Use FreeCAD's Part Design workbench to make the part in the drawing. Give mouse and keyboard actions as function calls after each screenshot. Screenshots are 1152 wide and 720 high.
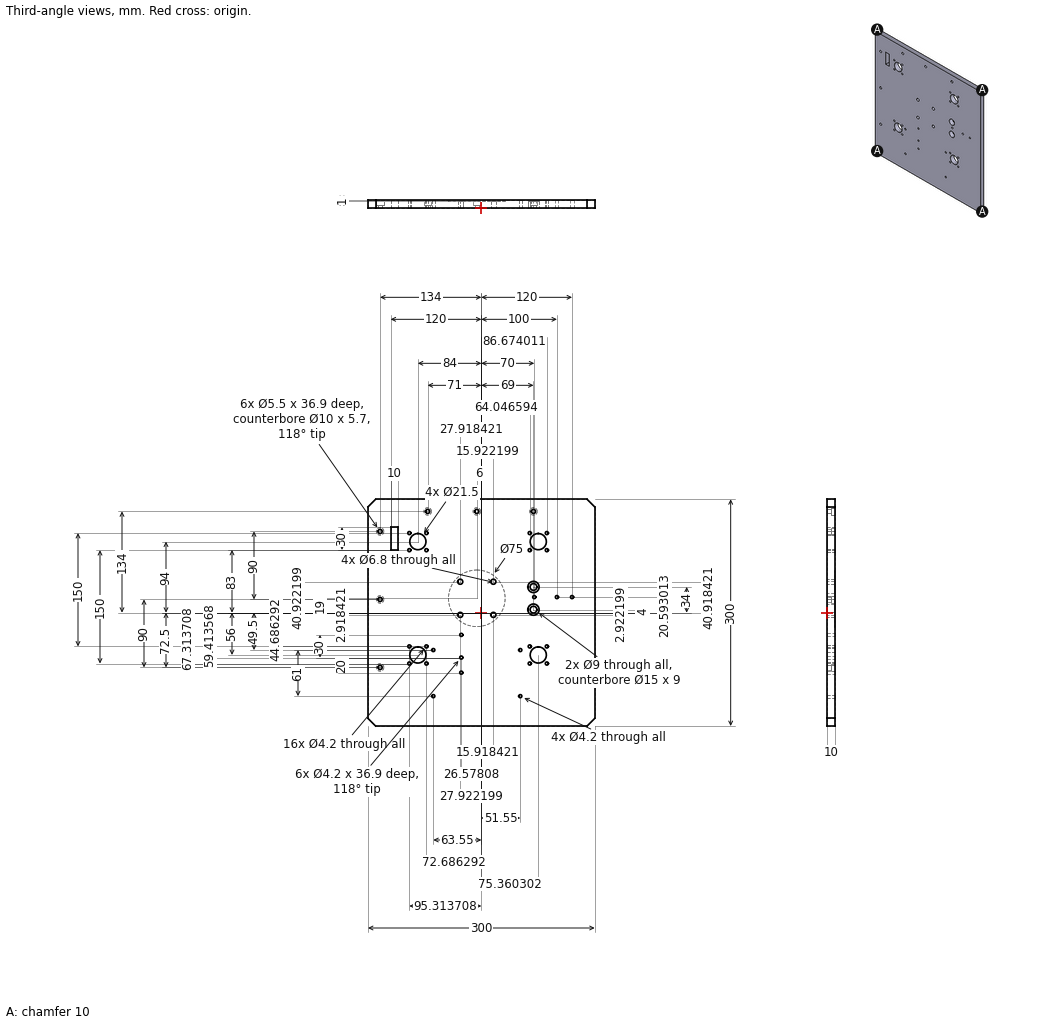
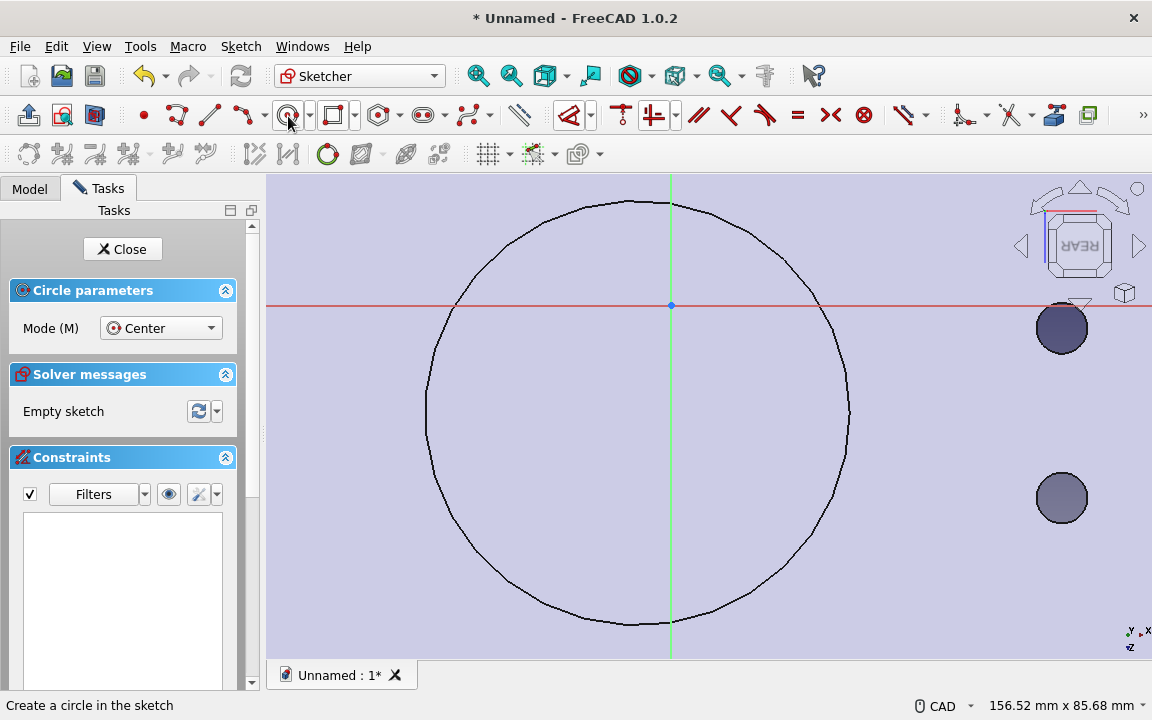
click(762, 537)
move(775, 524)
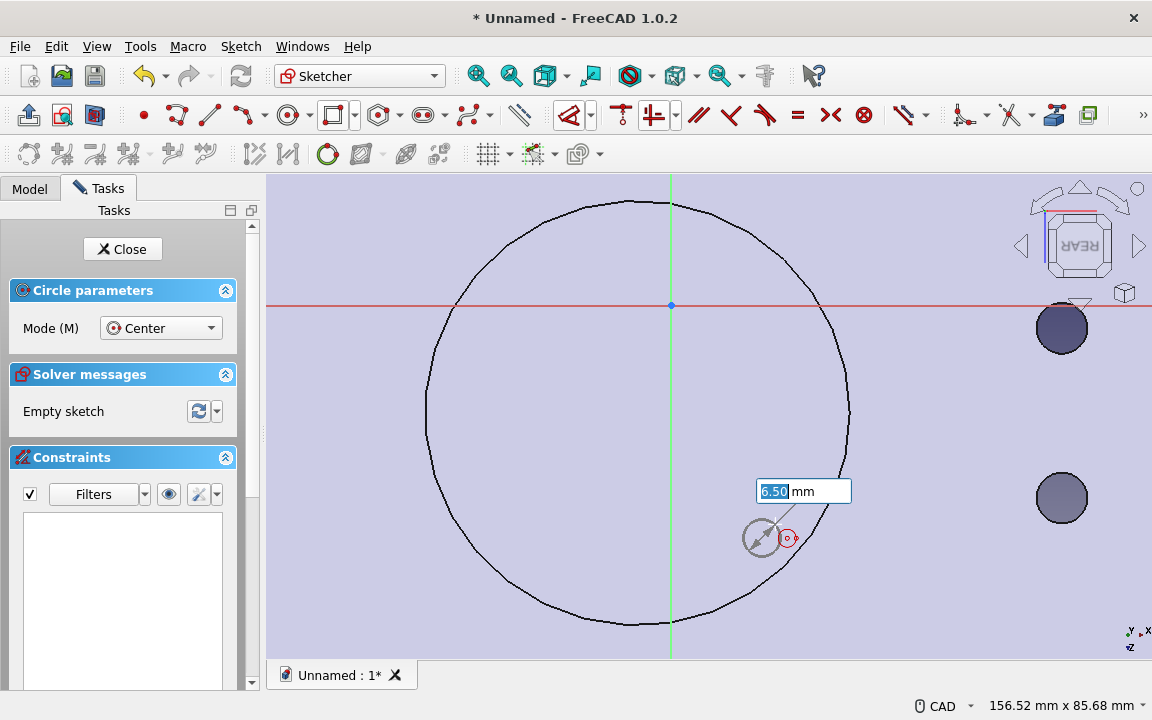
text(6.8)
key(Return)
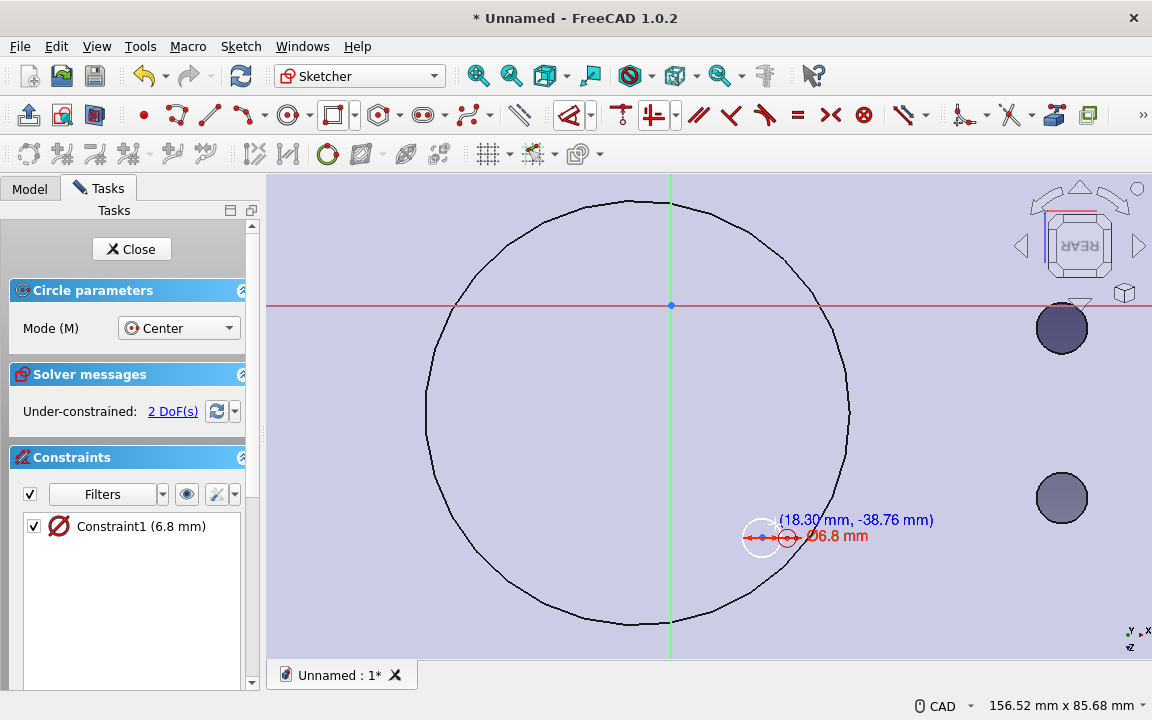
click(762, 289)
move(775, 275)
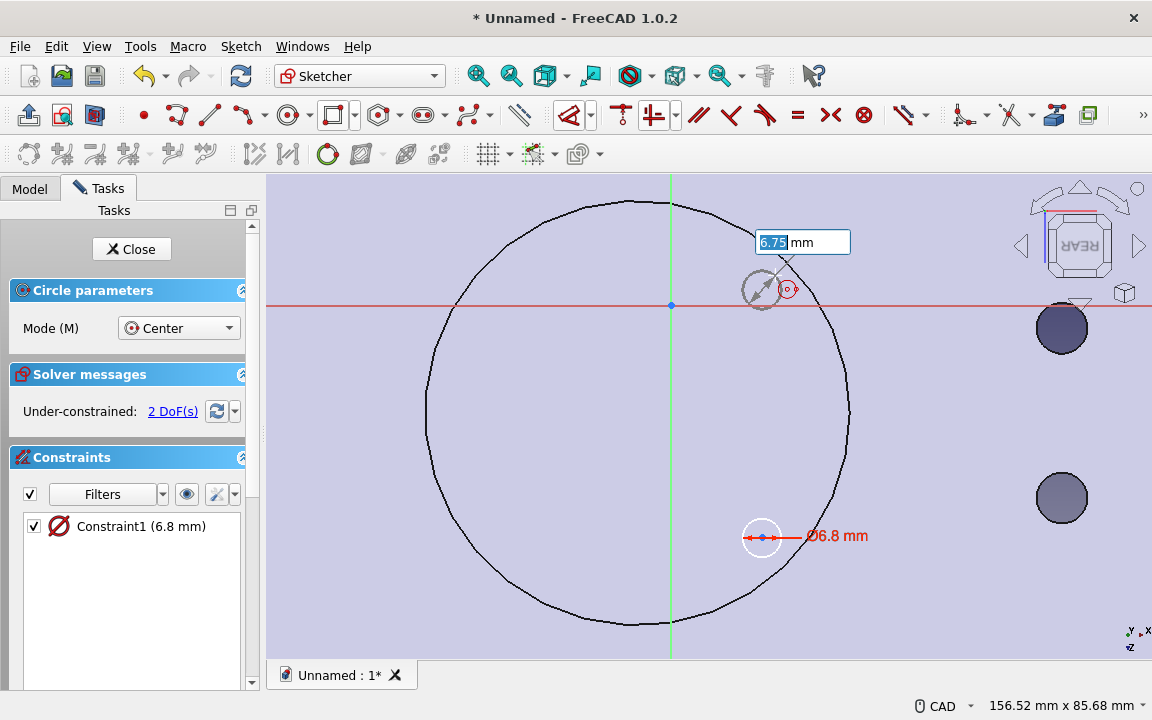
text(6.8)
key(Return)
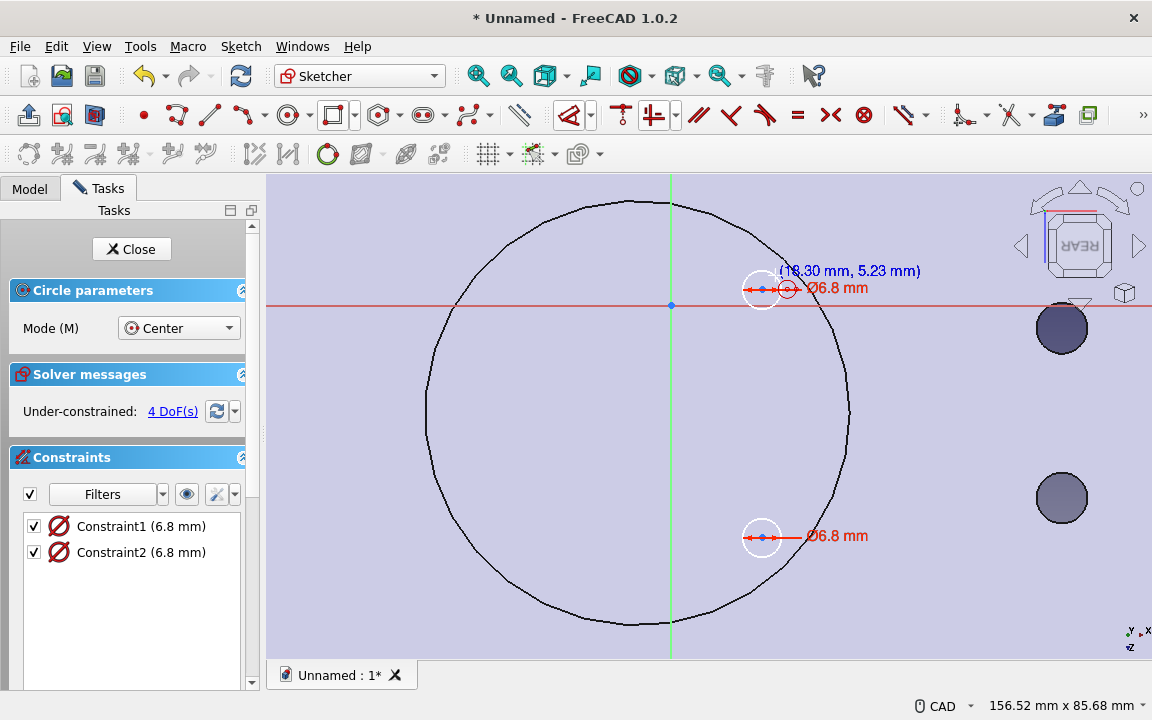
click(513, 289)
move(527, 275)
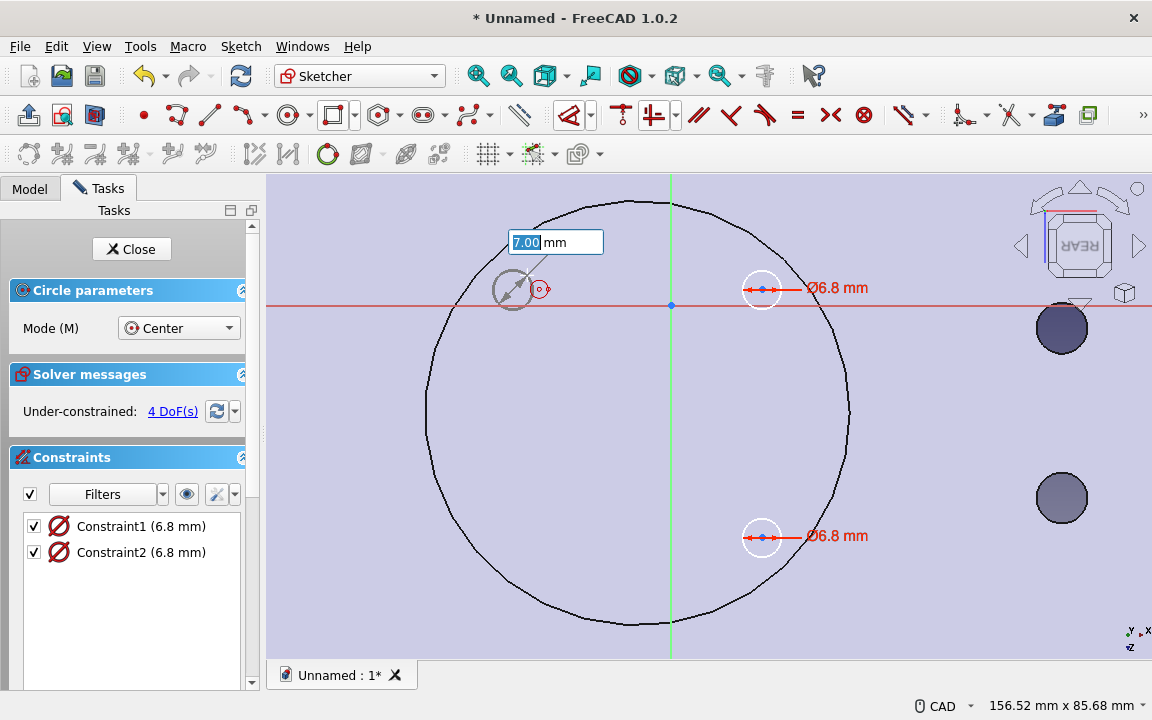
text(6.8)
key(Return)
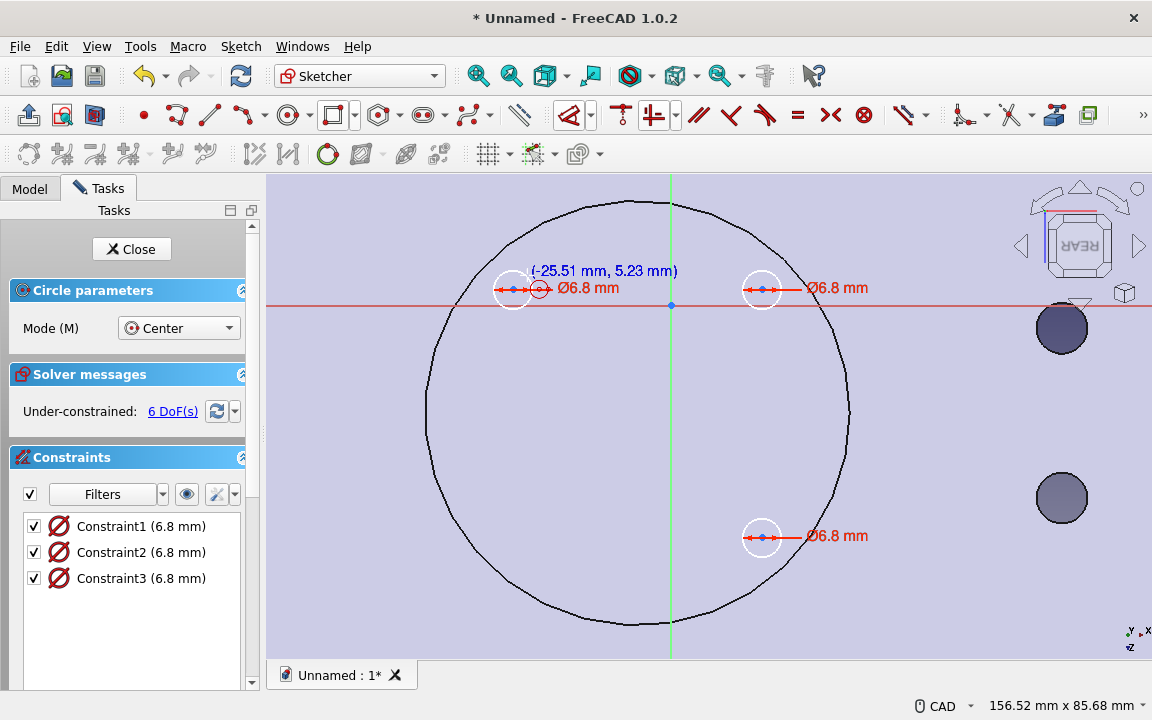
click(513, 537)
move(527, 524)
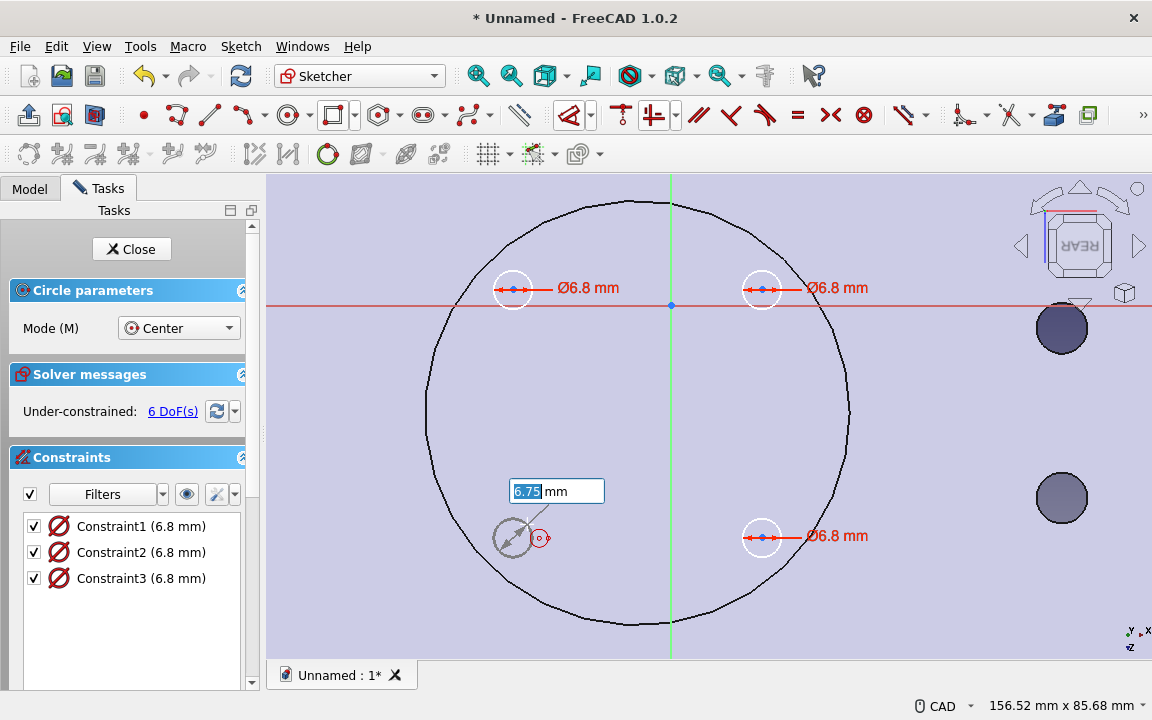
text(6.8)
key(Return)
key(Escape)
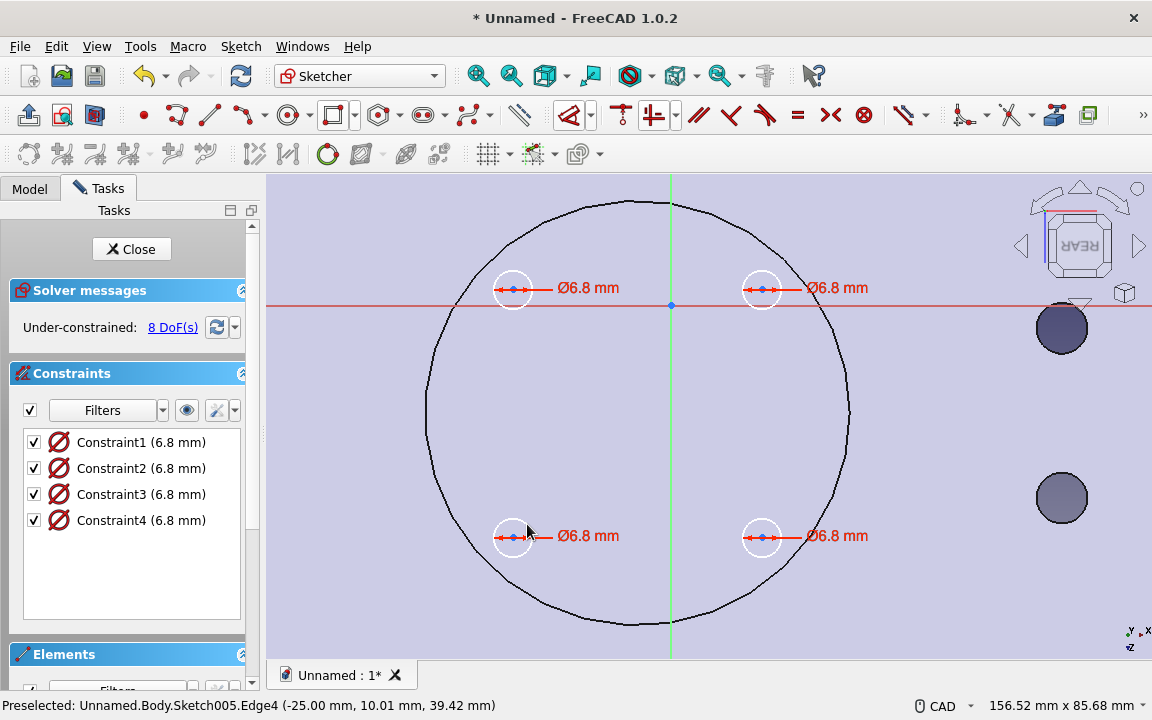
scroll(762, 290, up, 5)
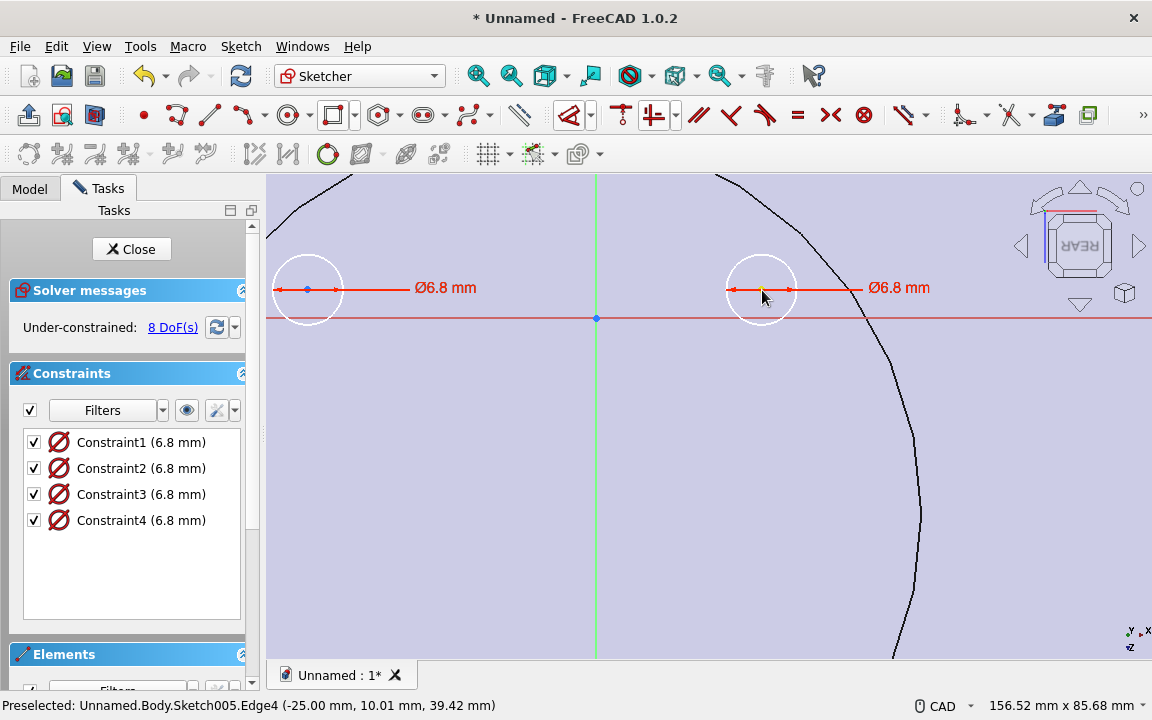
click(761, 290)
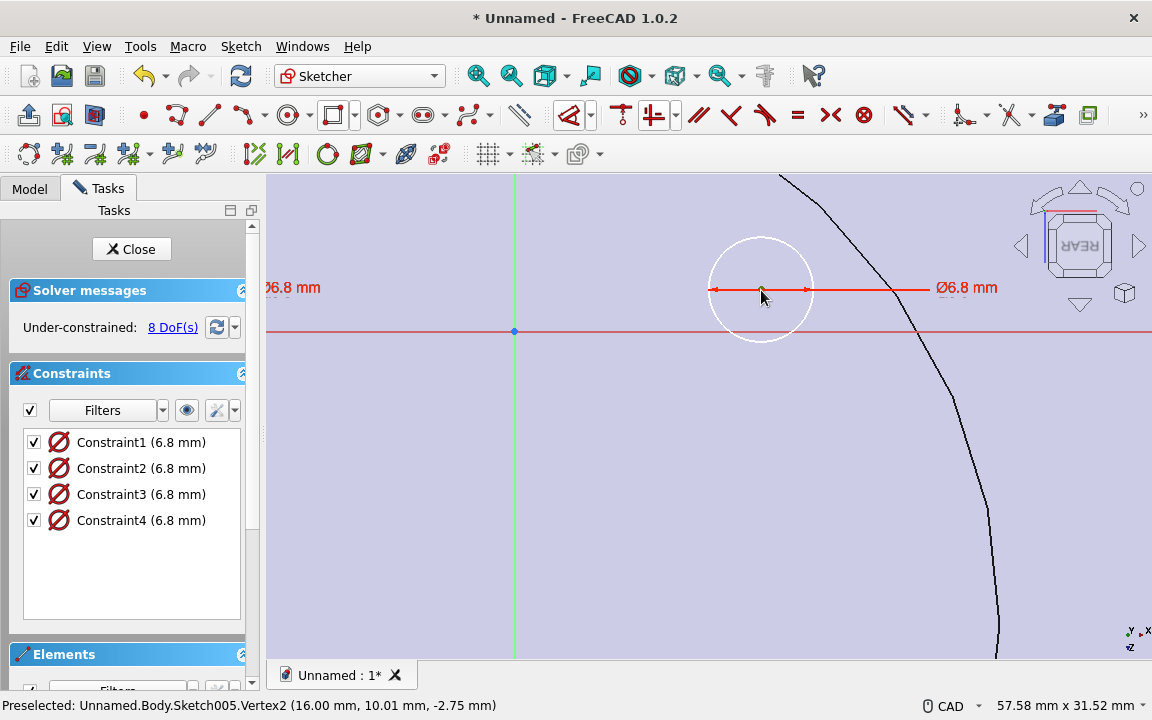
key(i)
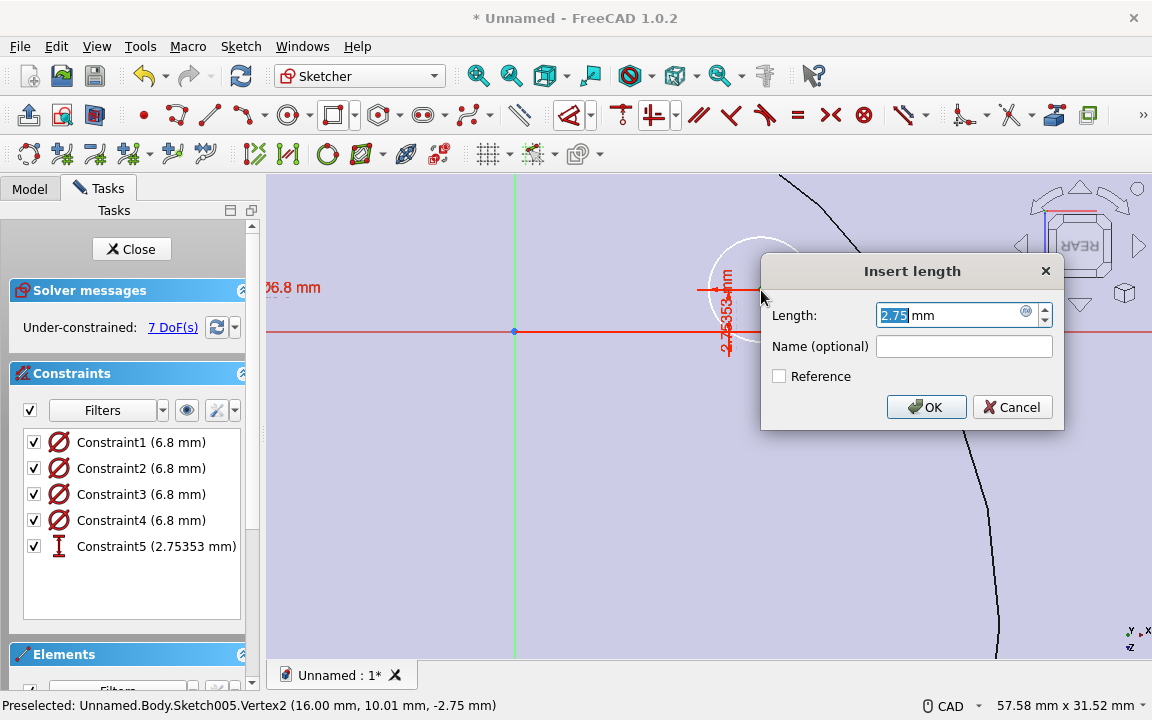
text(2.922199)
key(Return)